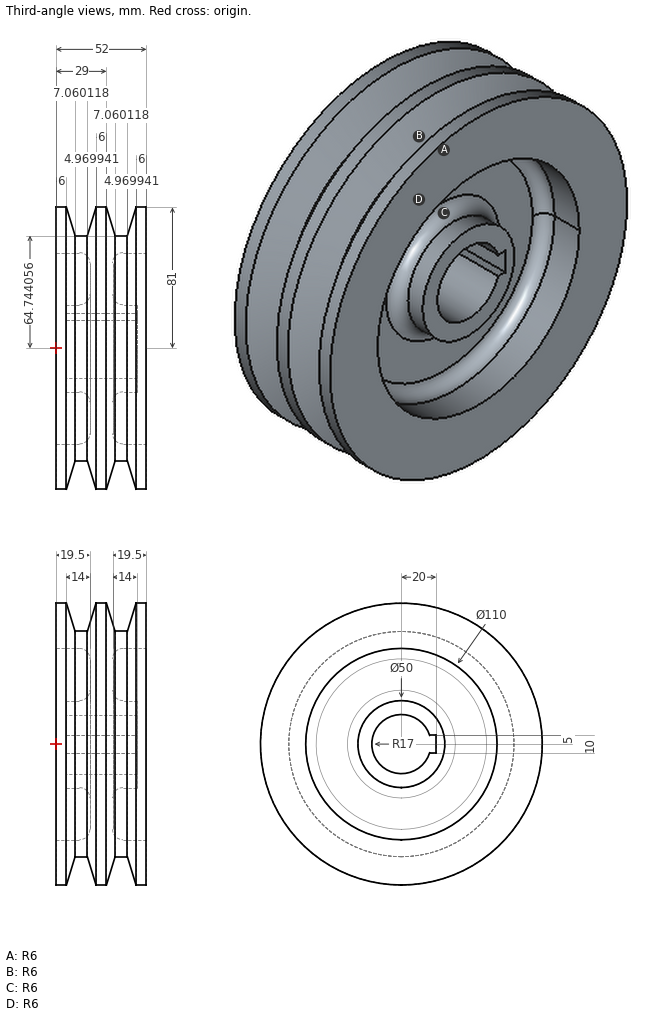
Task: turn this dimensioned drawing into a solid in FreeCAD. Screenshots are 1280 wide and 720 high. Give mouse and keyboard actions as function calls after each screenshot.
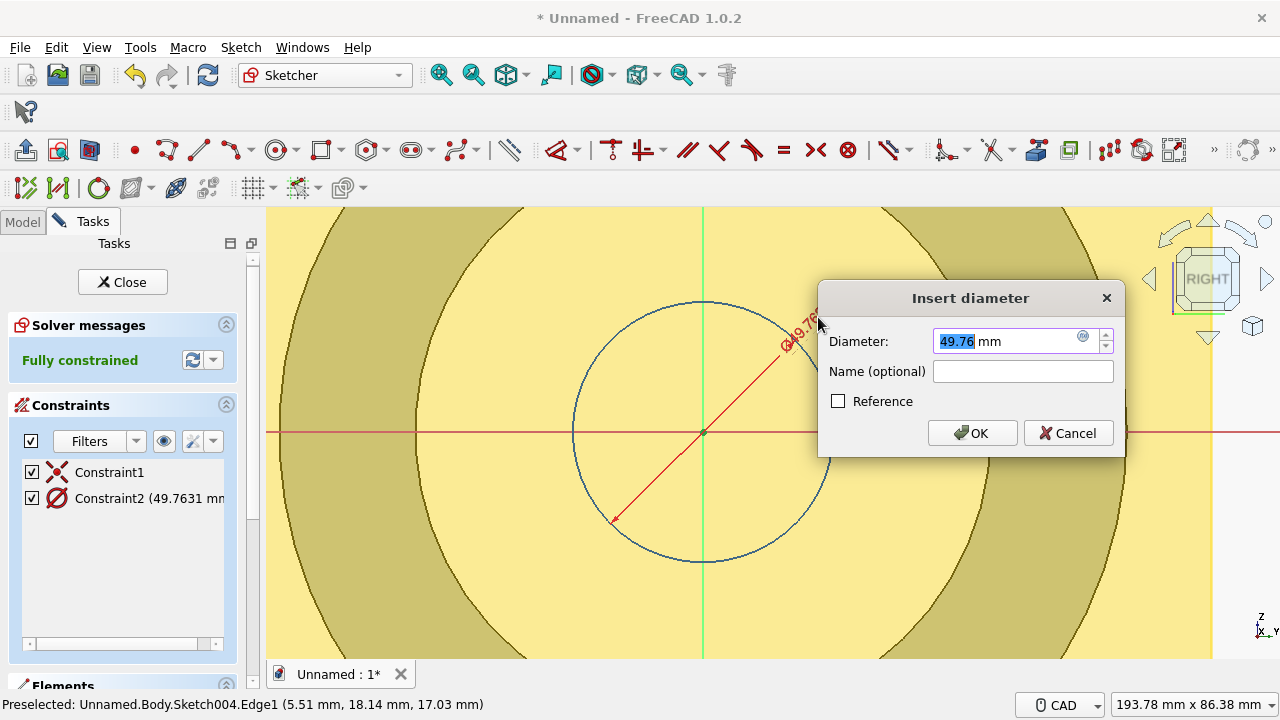
text(50)
key(Return)
key(Escape)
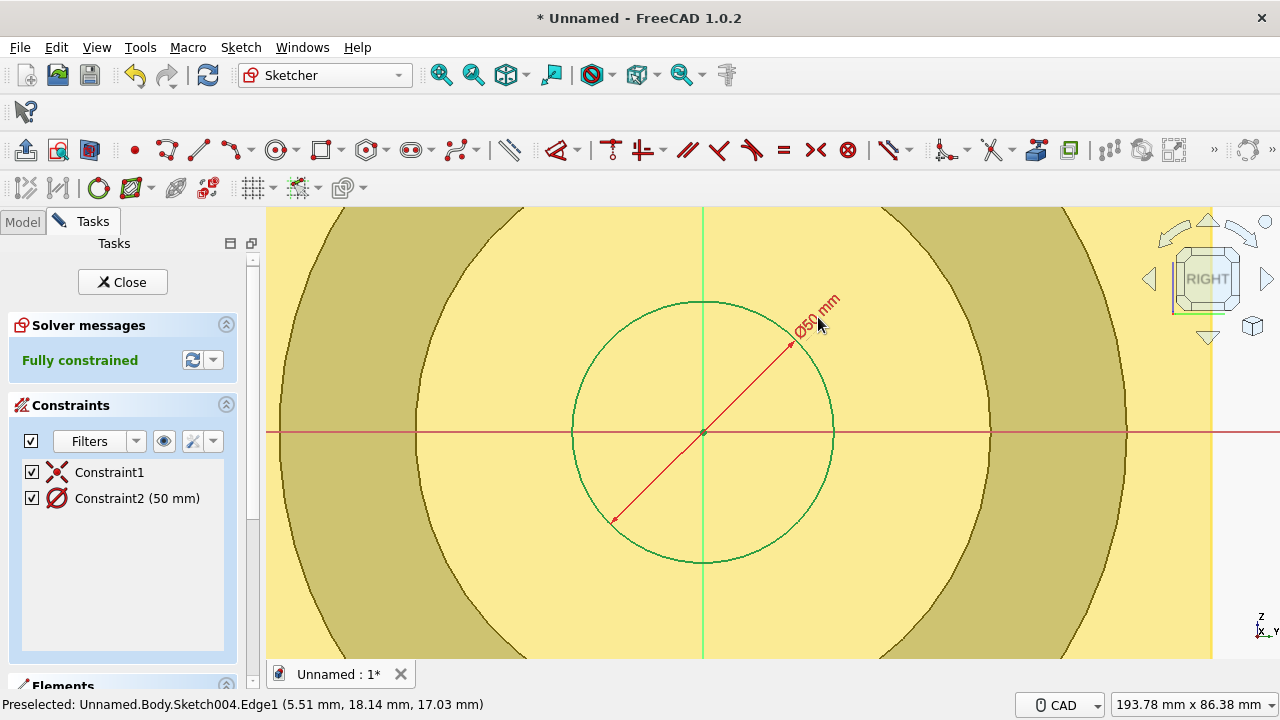
click(123, 282)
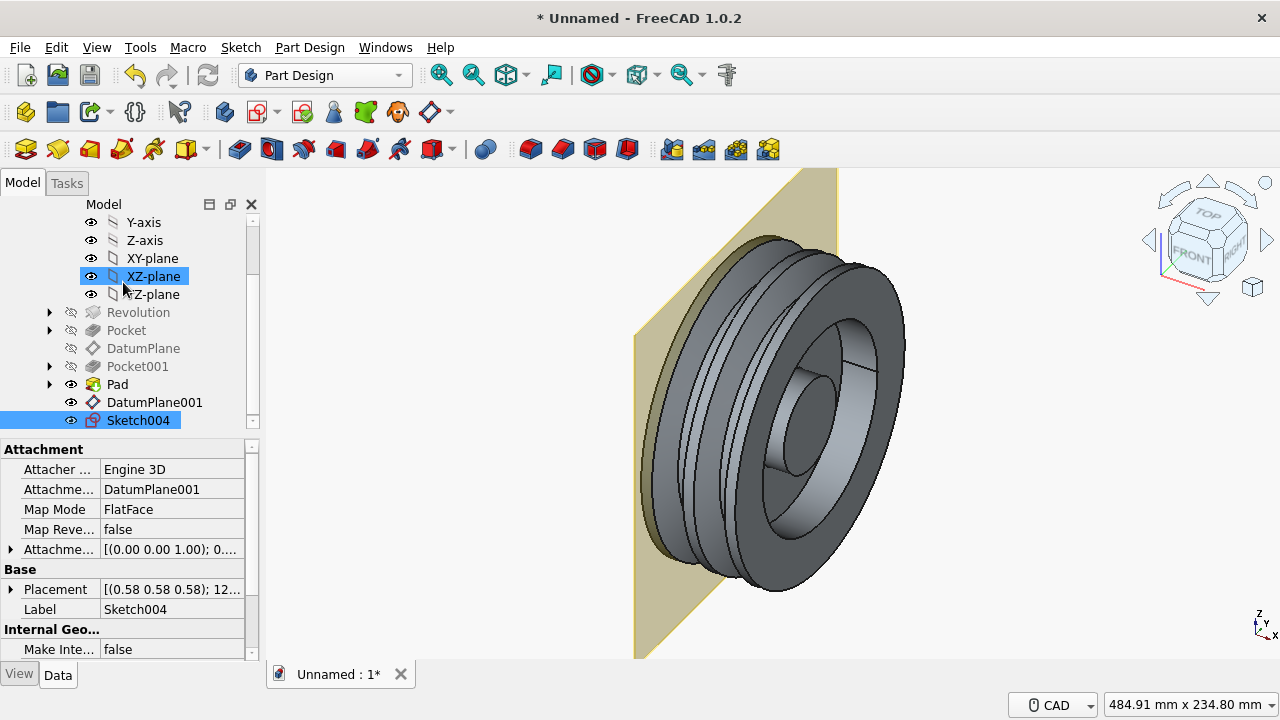
click(26, 150)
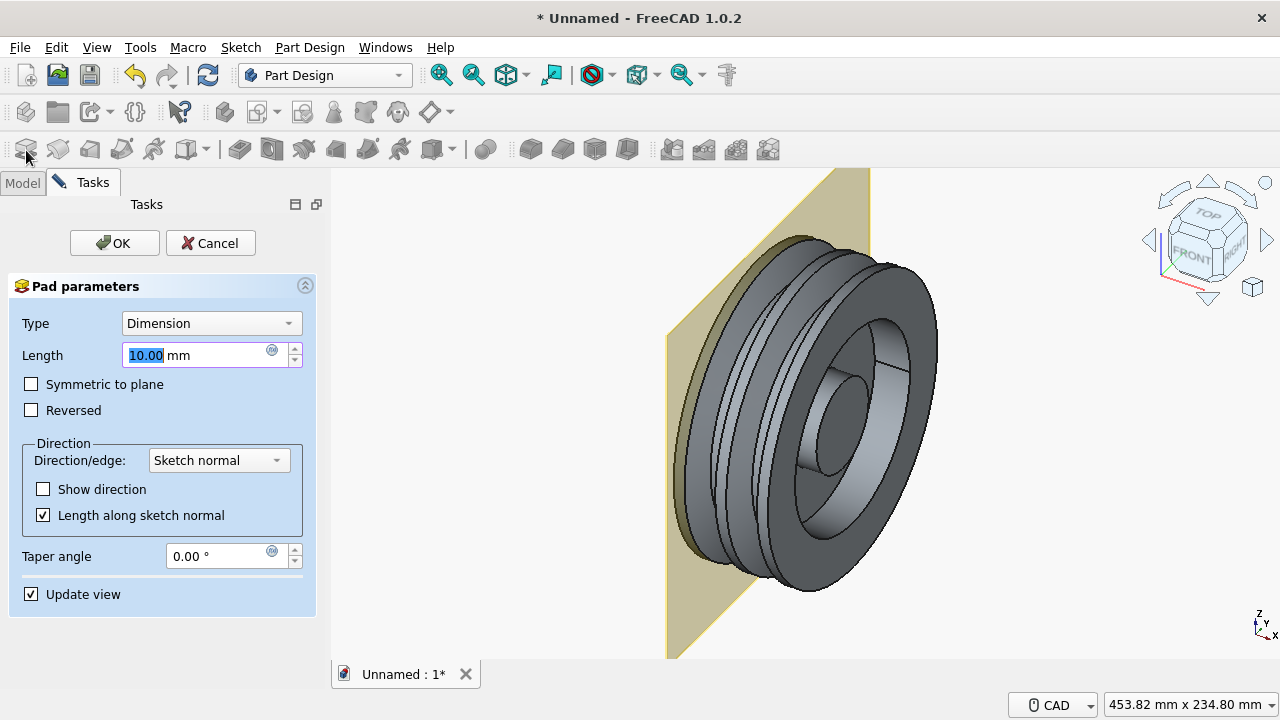
text(14)
key(Tab)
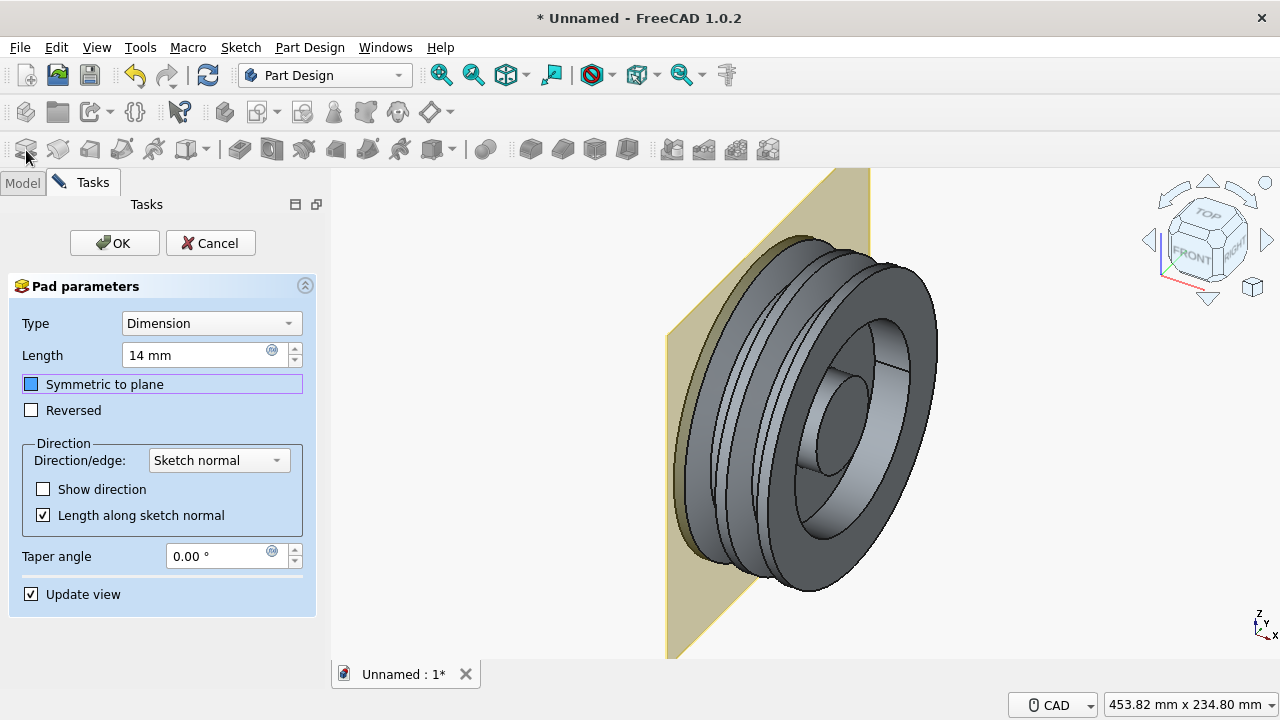
click(115, 243)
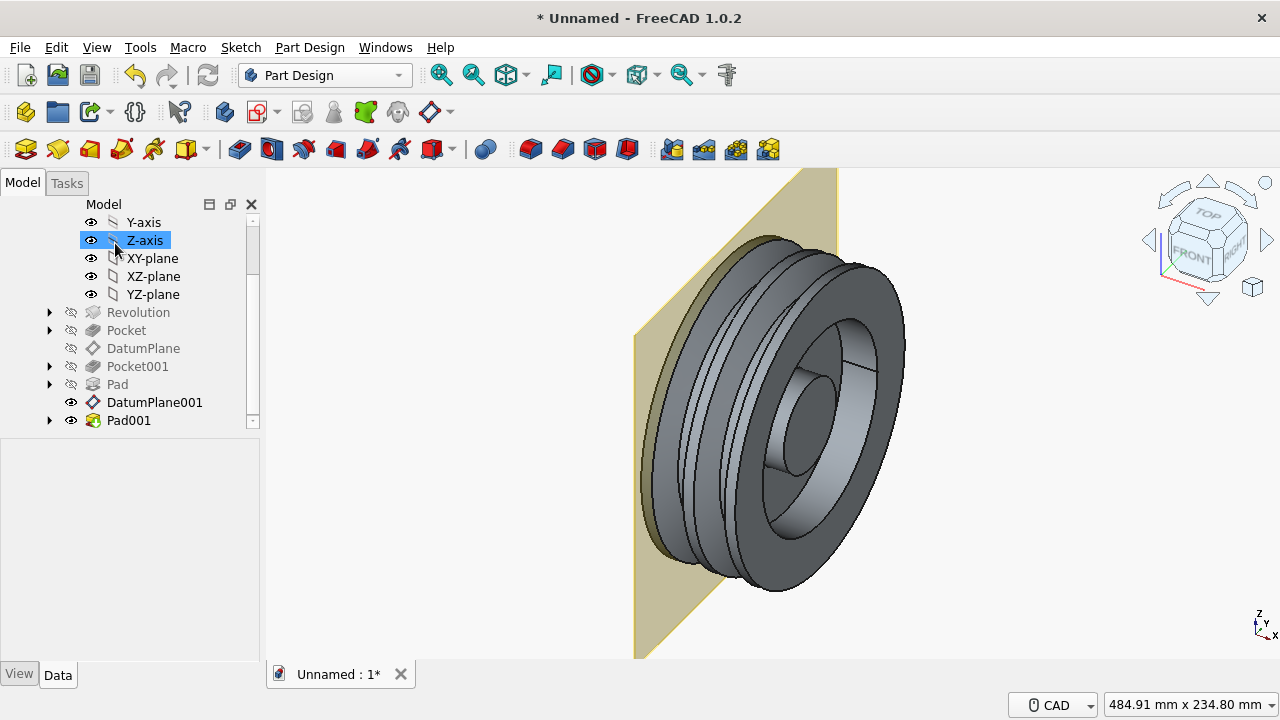
click(116, 402)
key(space)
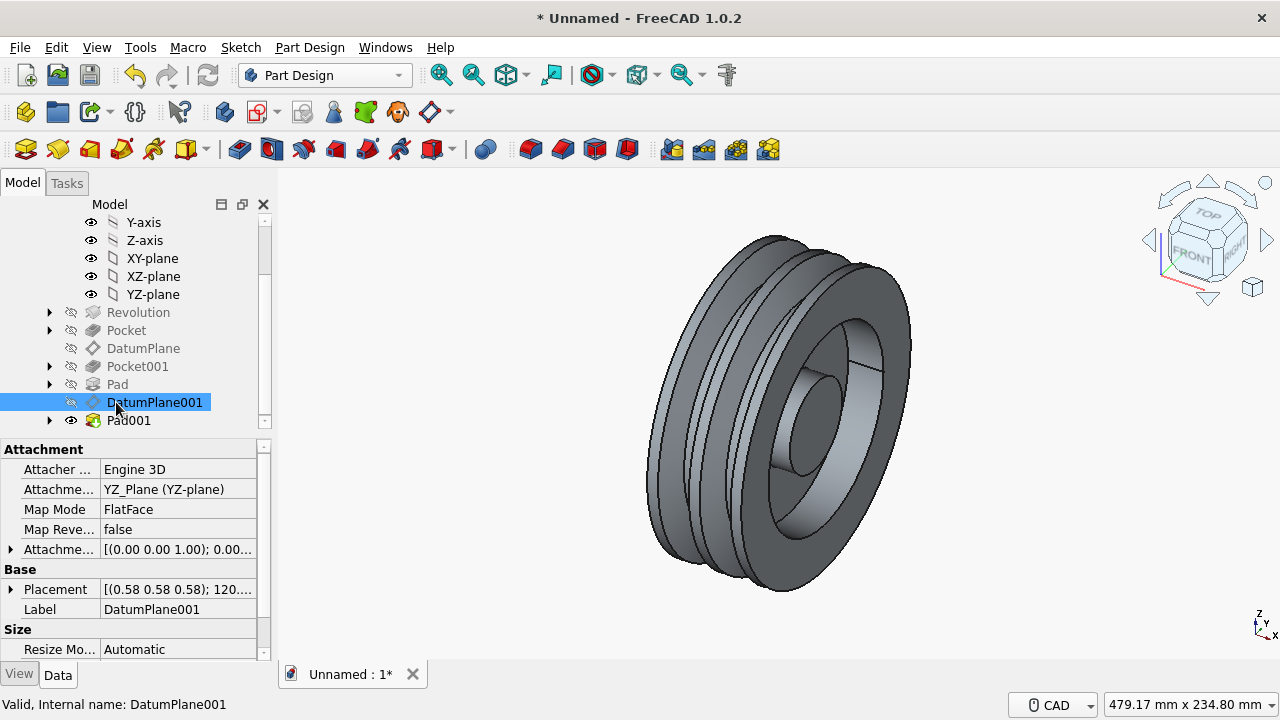
key(6)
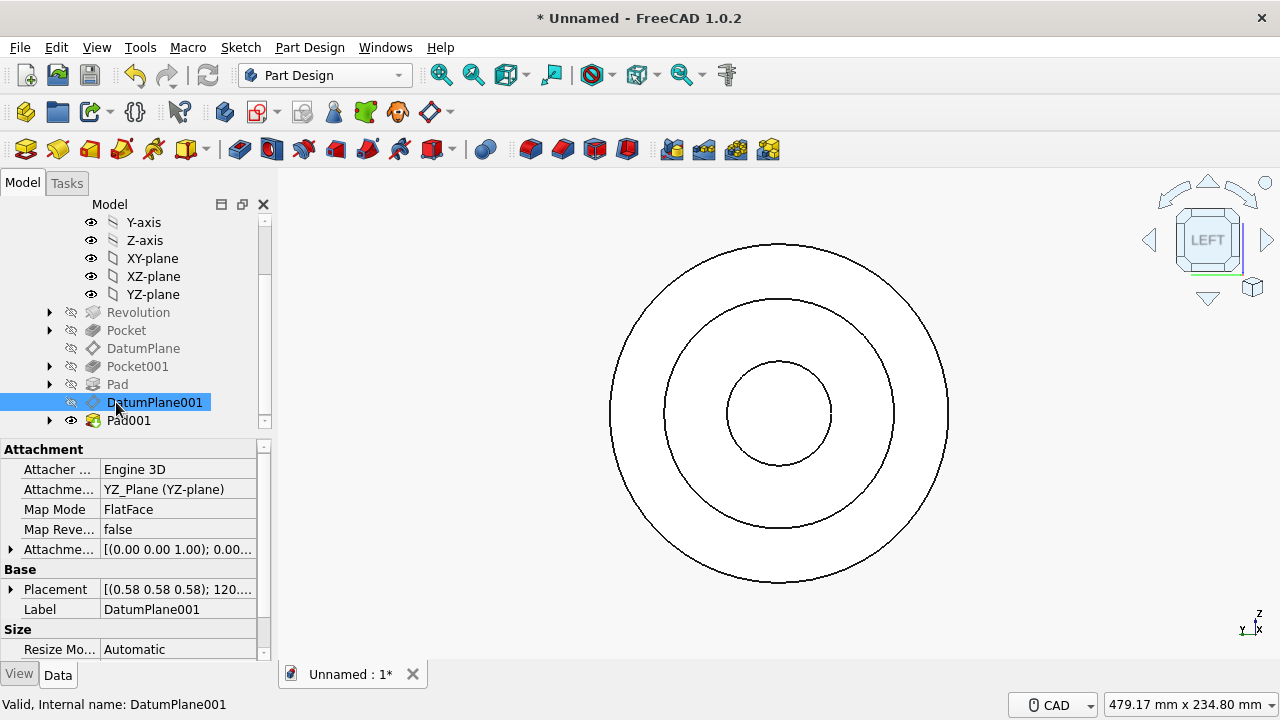
click(779, 412)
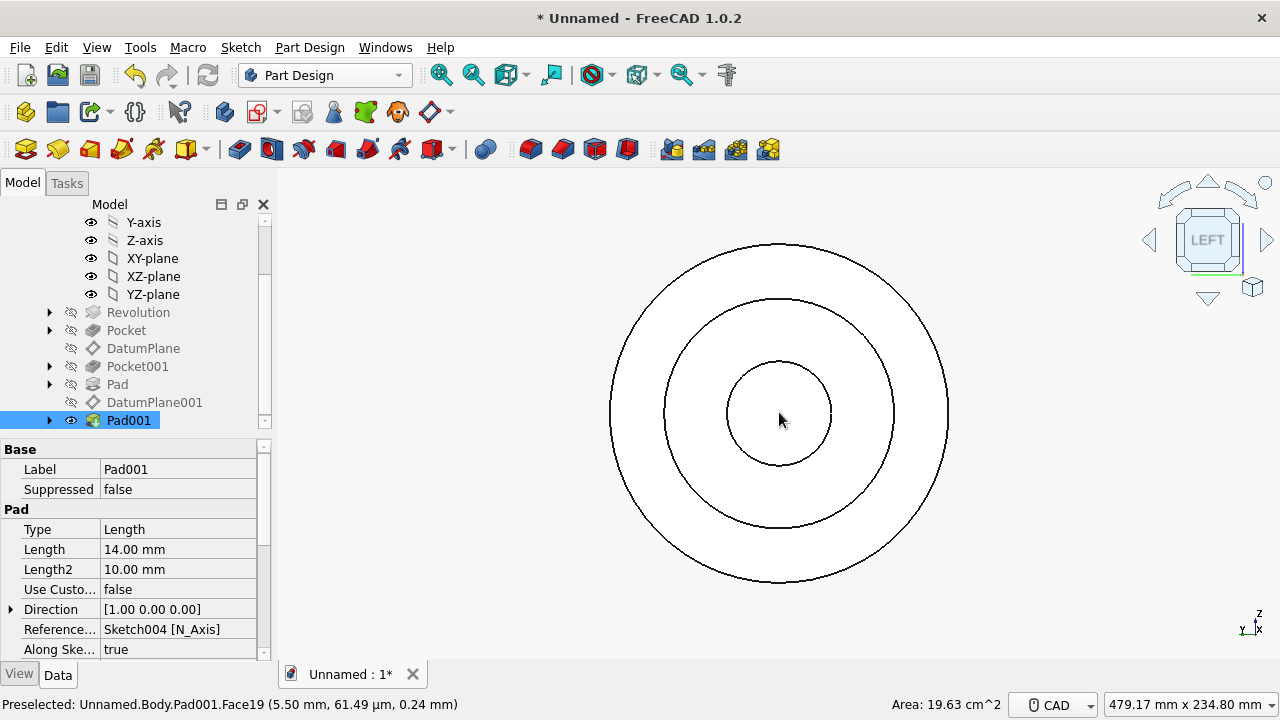
click(258, 112)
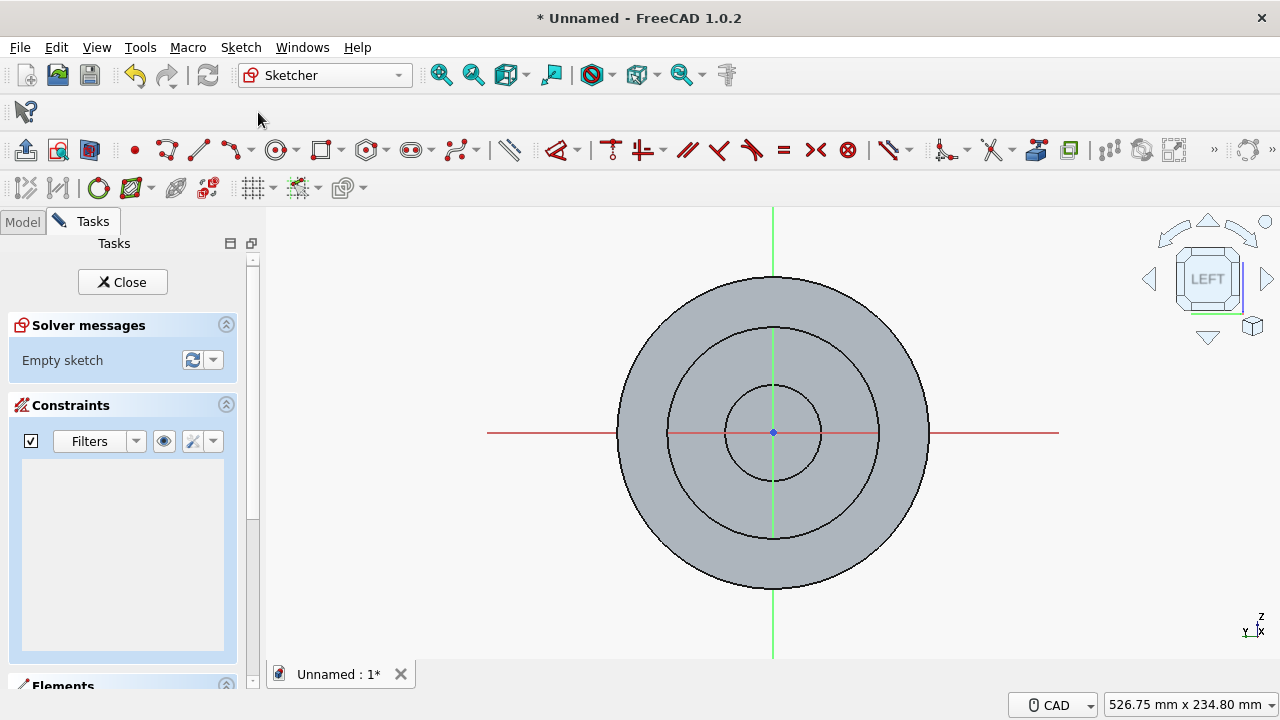
click(90, 150)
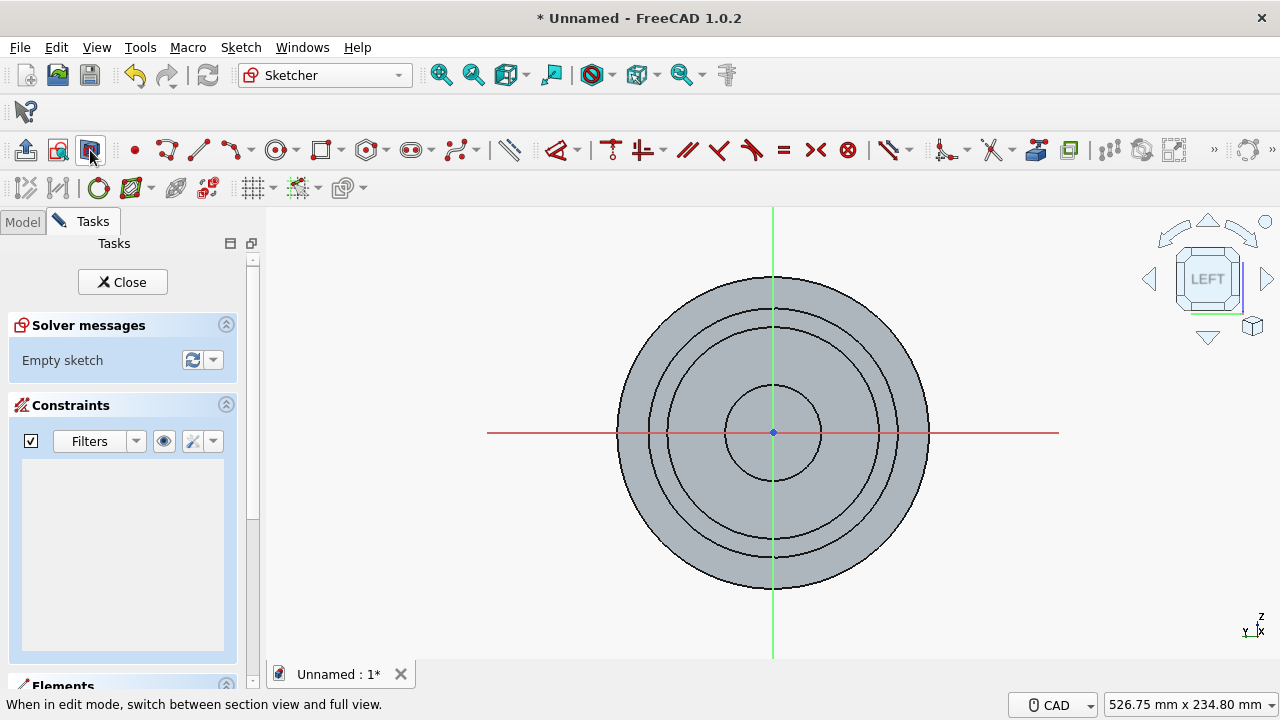
scroll(781, 433, up, 10)